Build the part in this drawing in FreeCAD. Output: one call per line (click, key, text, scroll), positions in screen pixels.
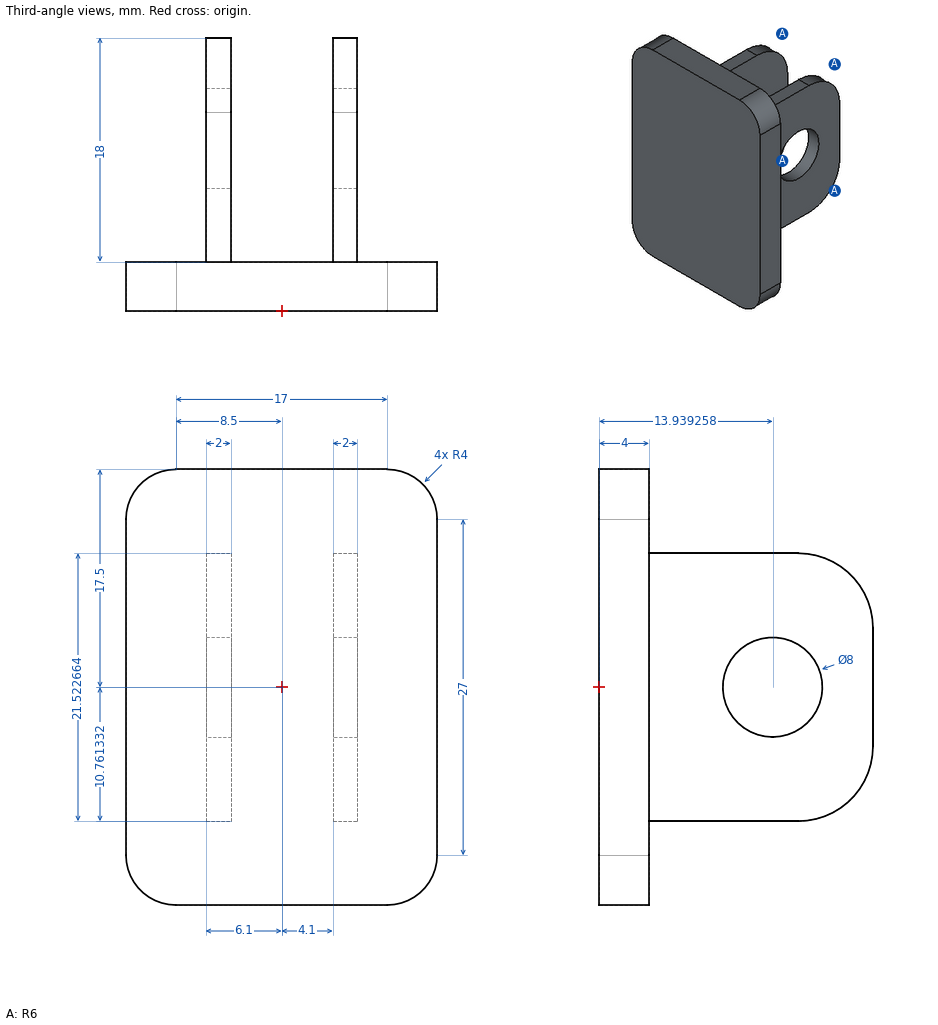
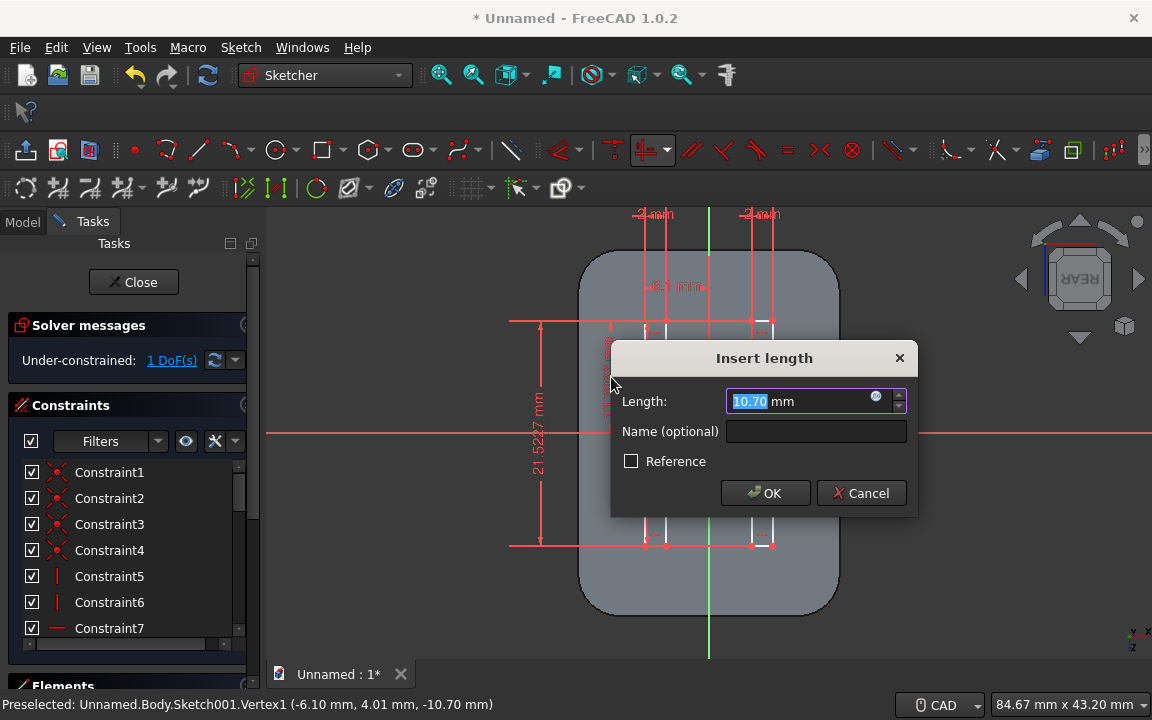
text(10.761332)
key(Return)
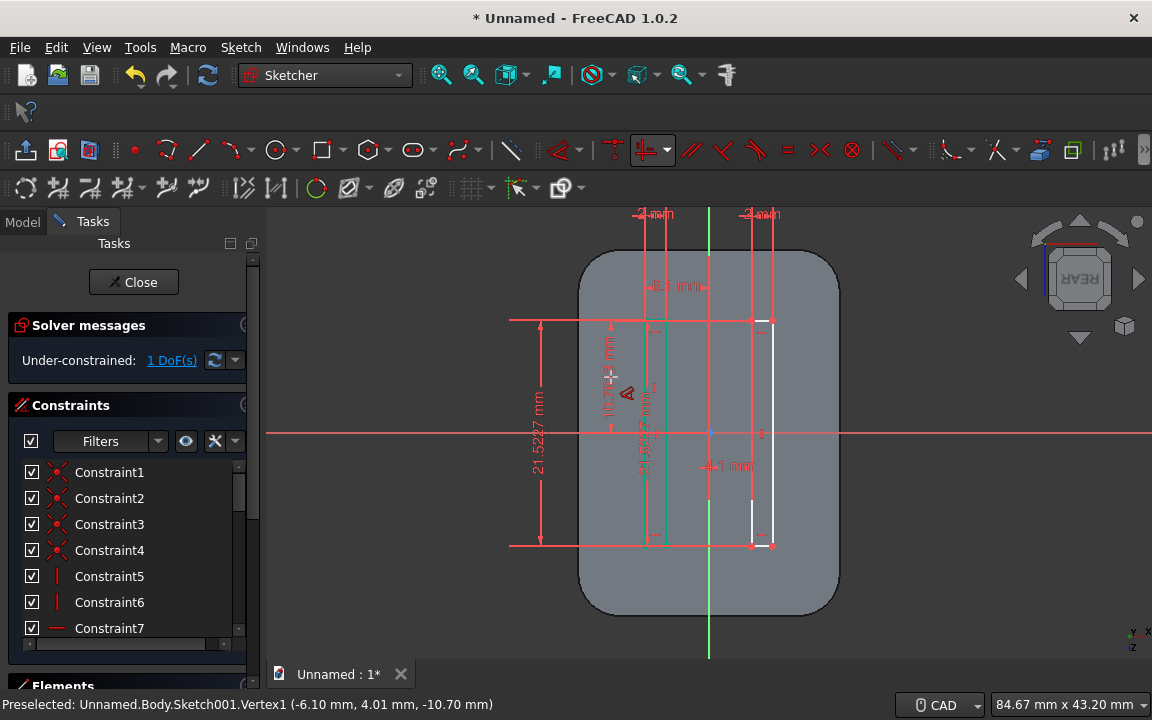
click(752, 321)
click(786, 377)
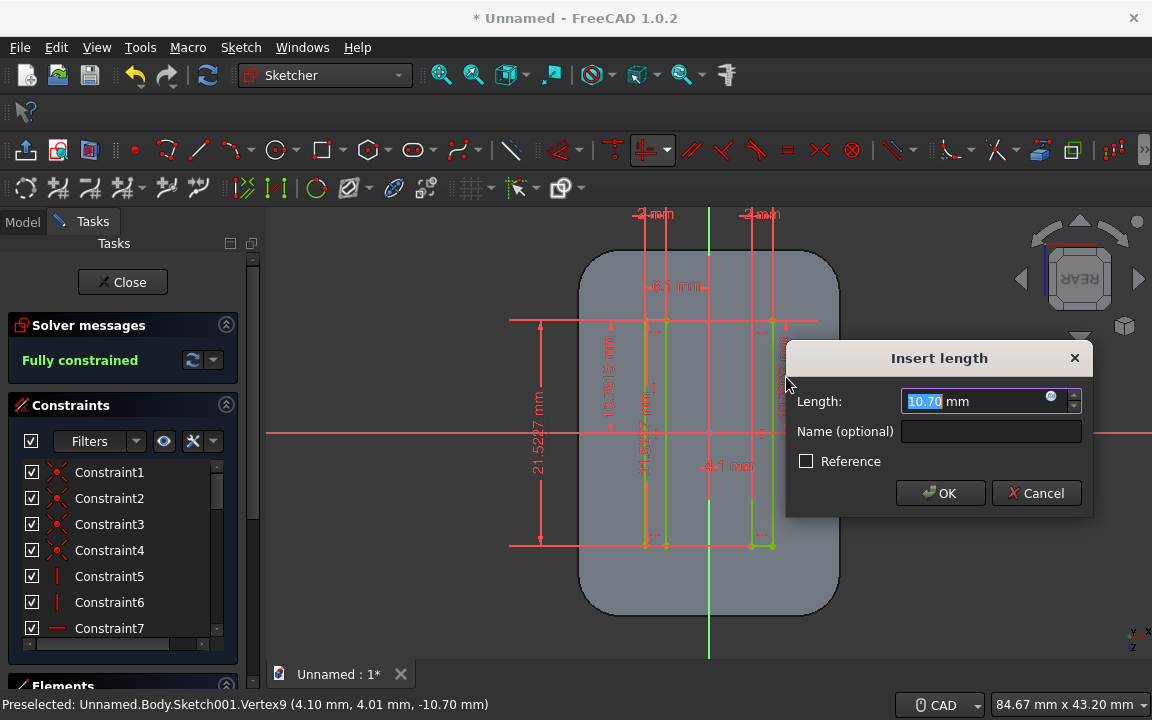
text(10.761332)
key(Return)
key(Escape)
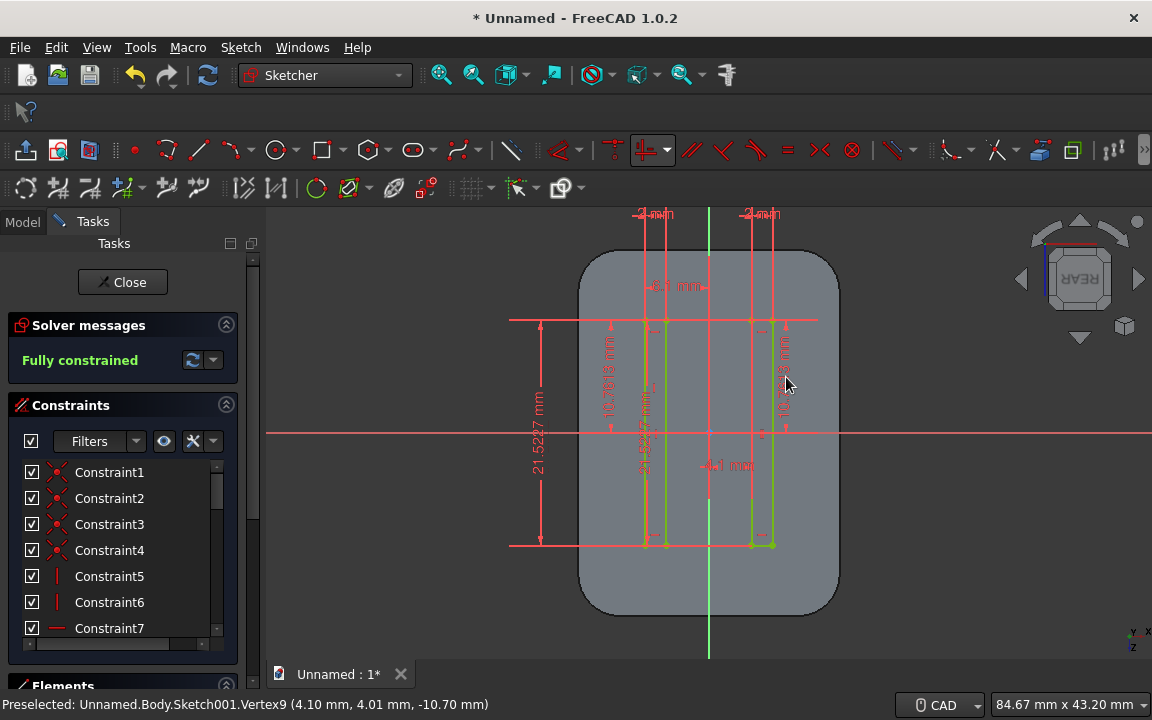
click(123, 282)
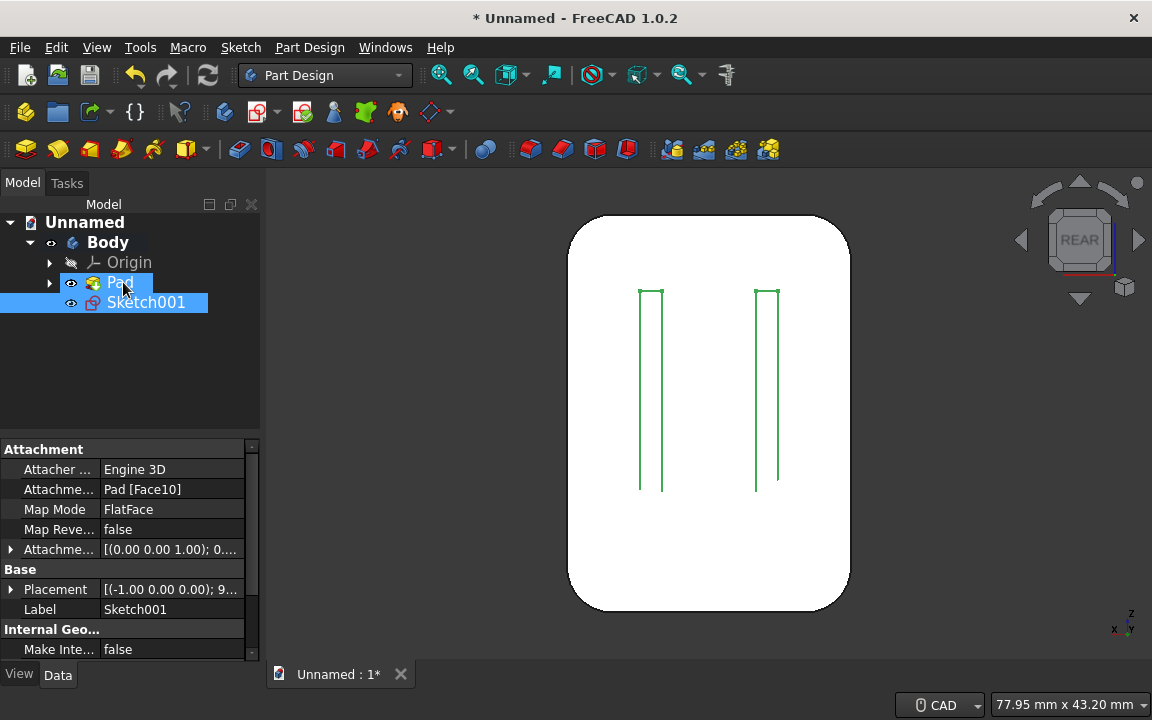
click(26, 150)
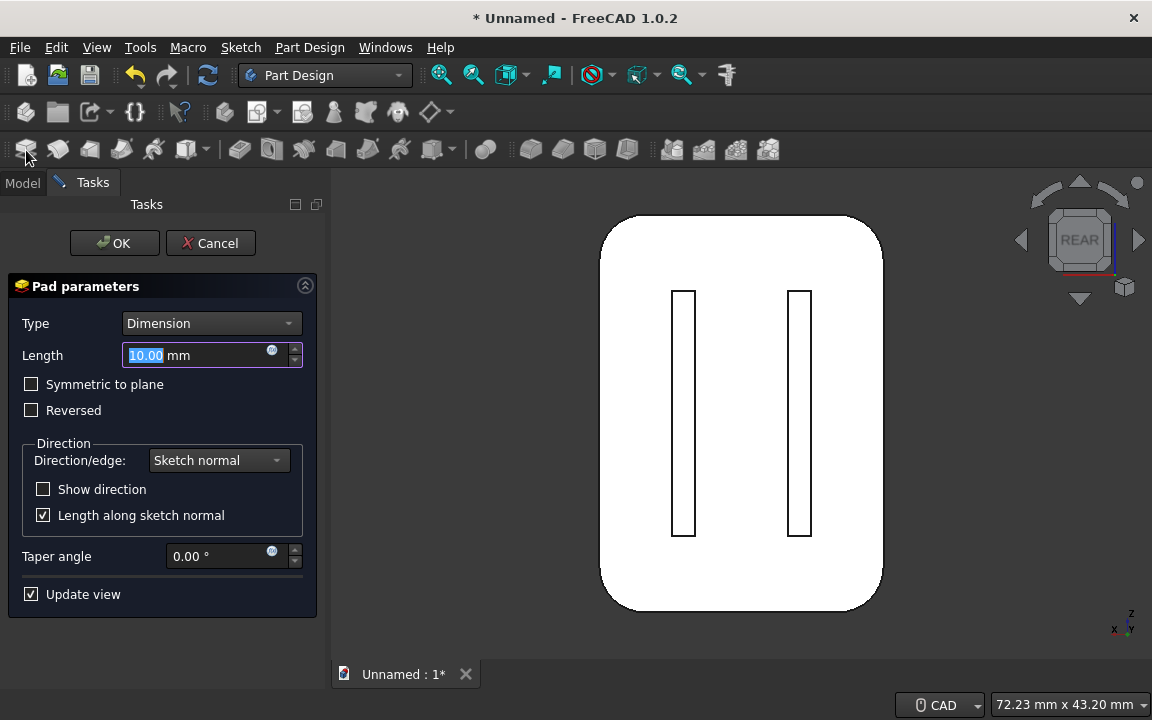
text(18)
key(Tab)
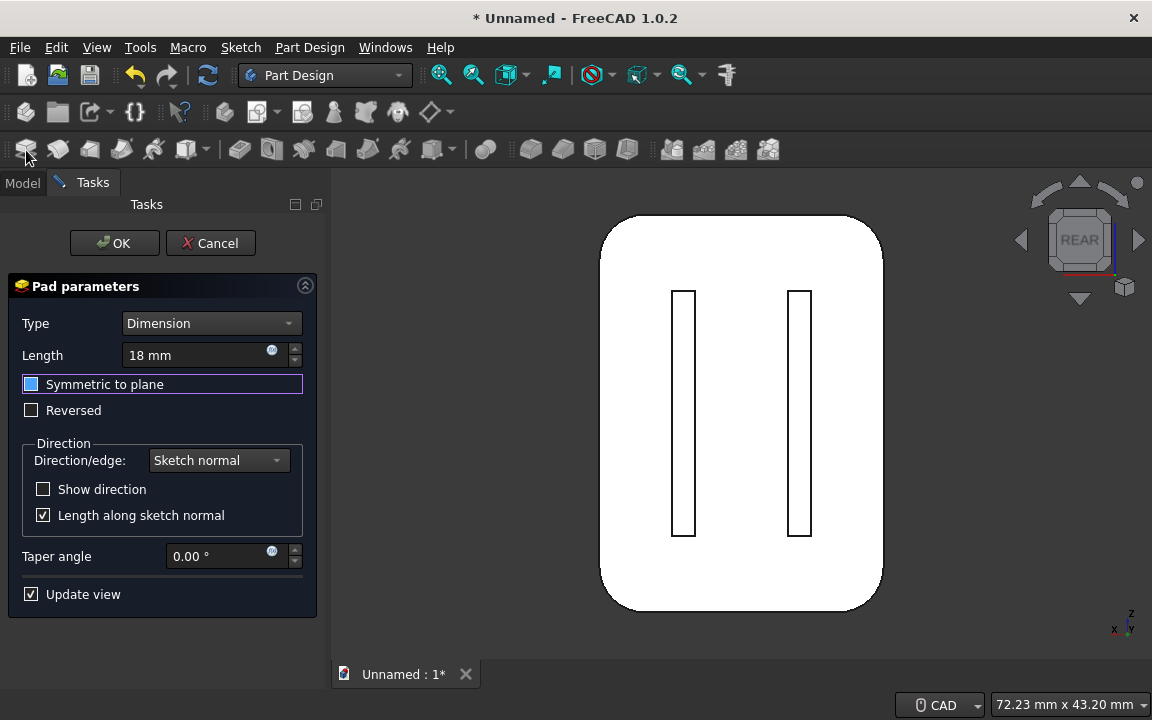
click(115, 243)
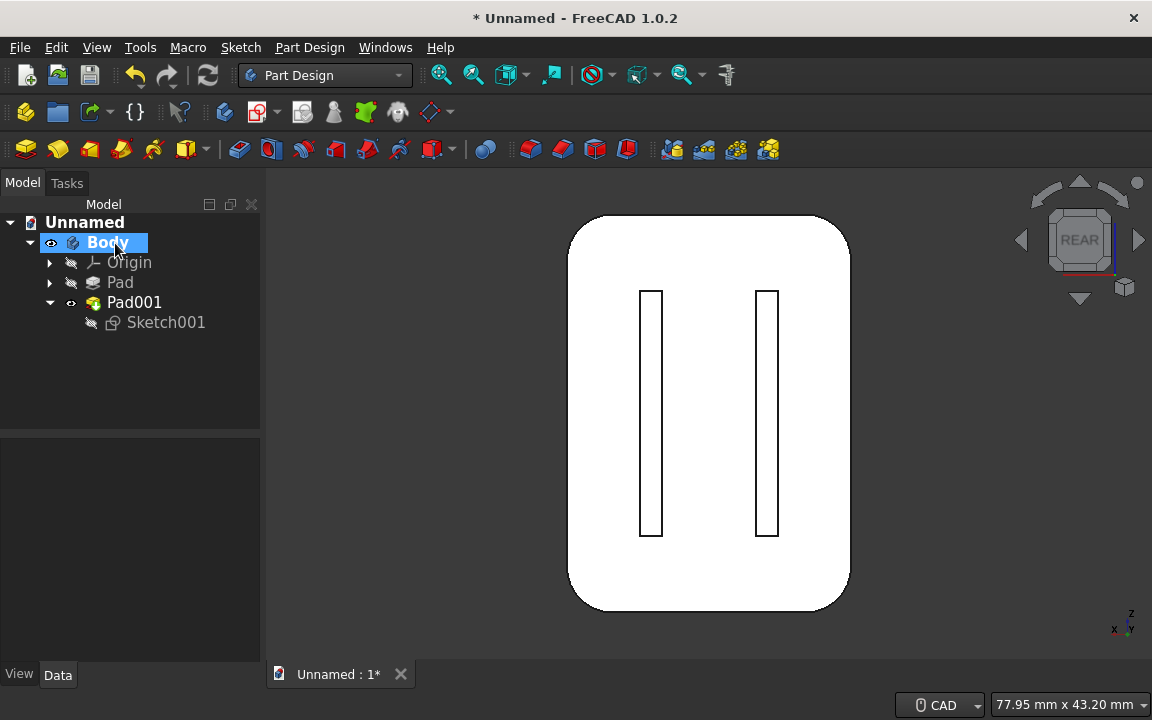
click(651, 535)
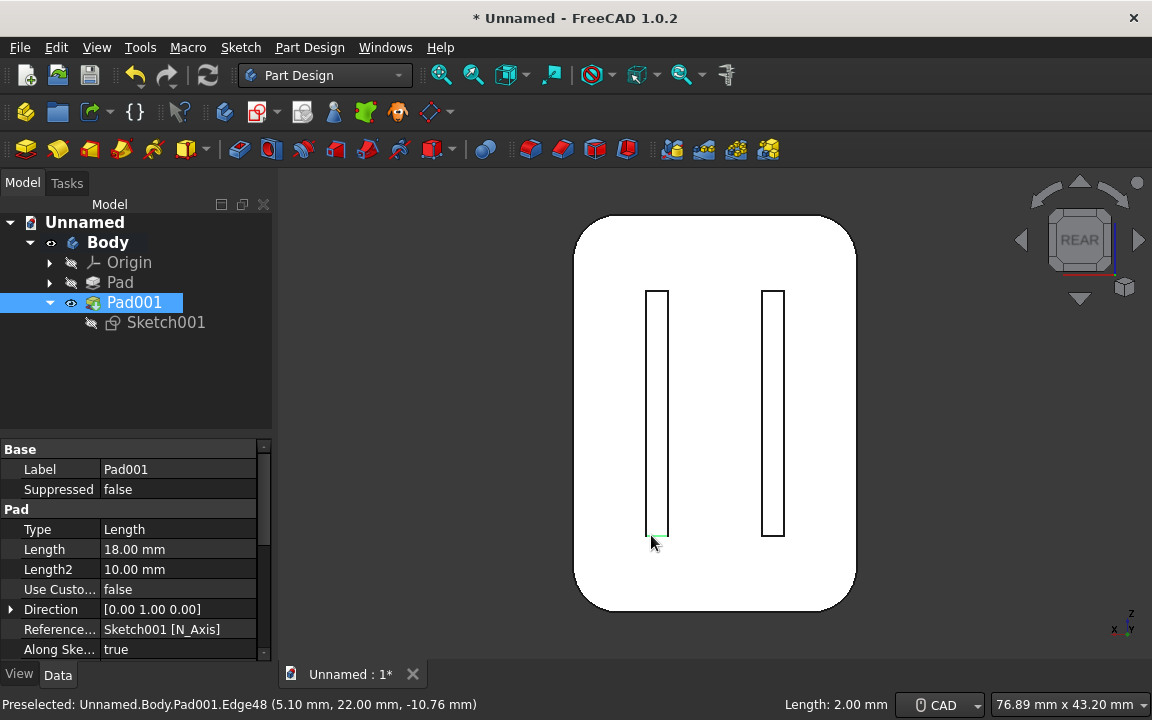
click(773, 535, ctrl)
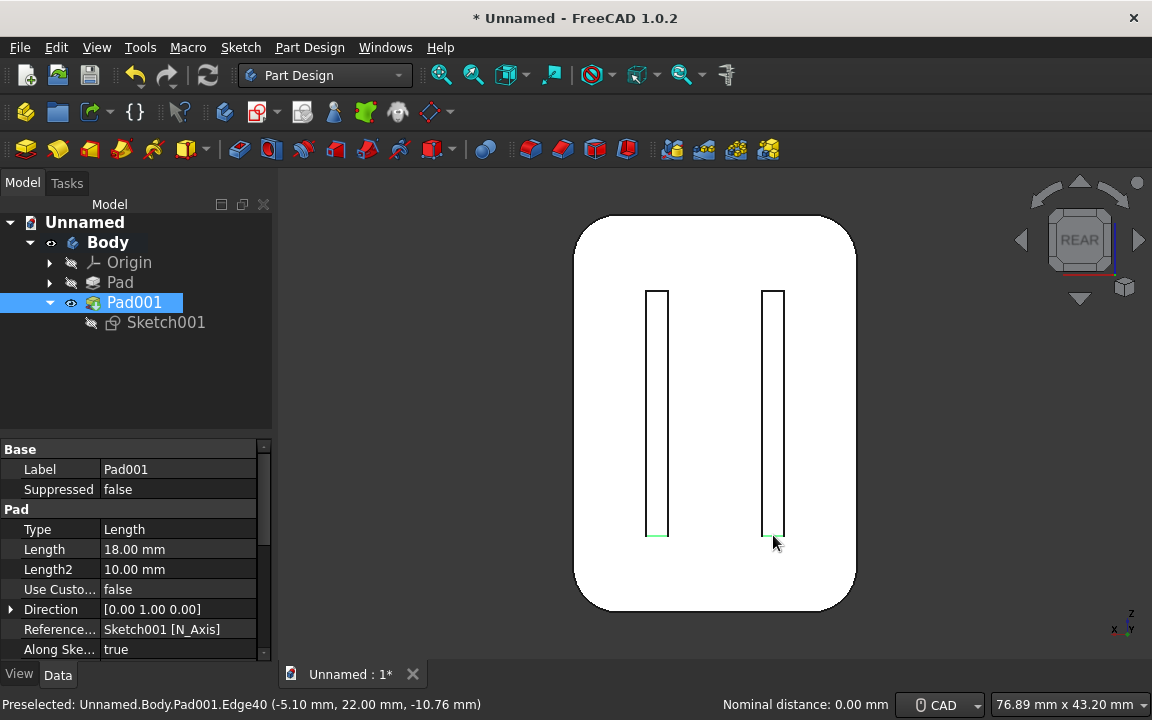
key(0)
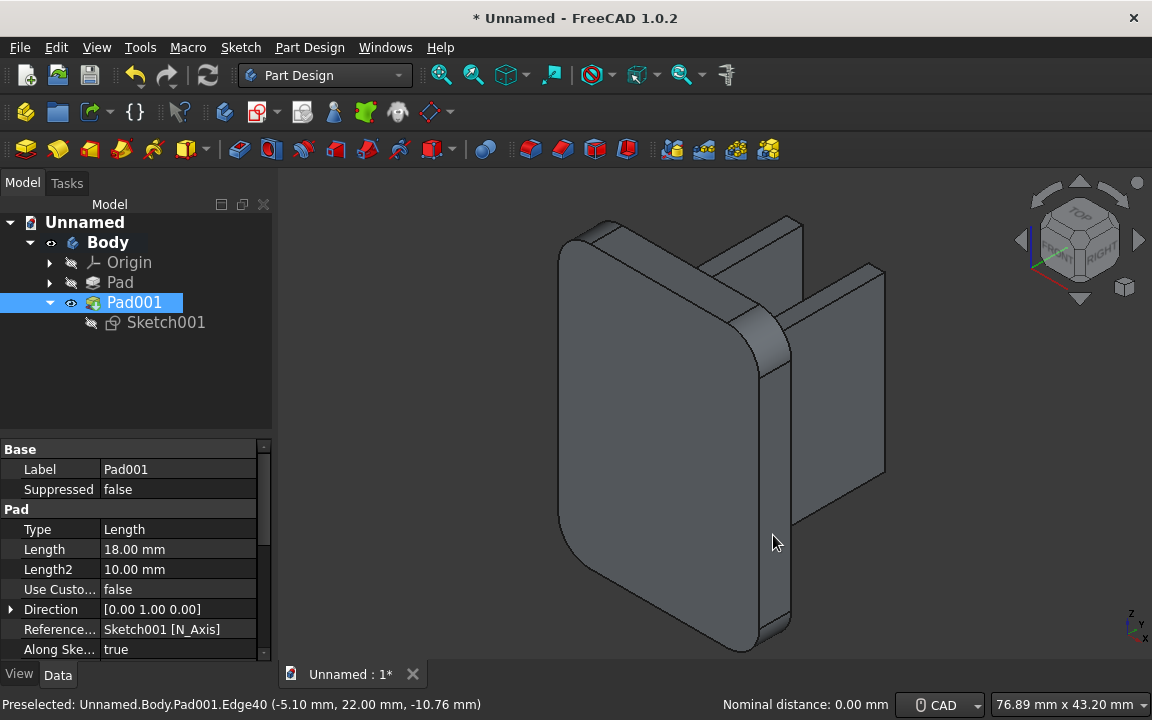
click(442, 76)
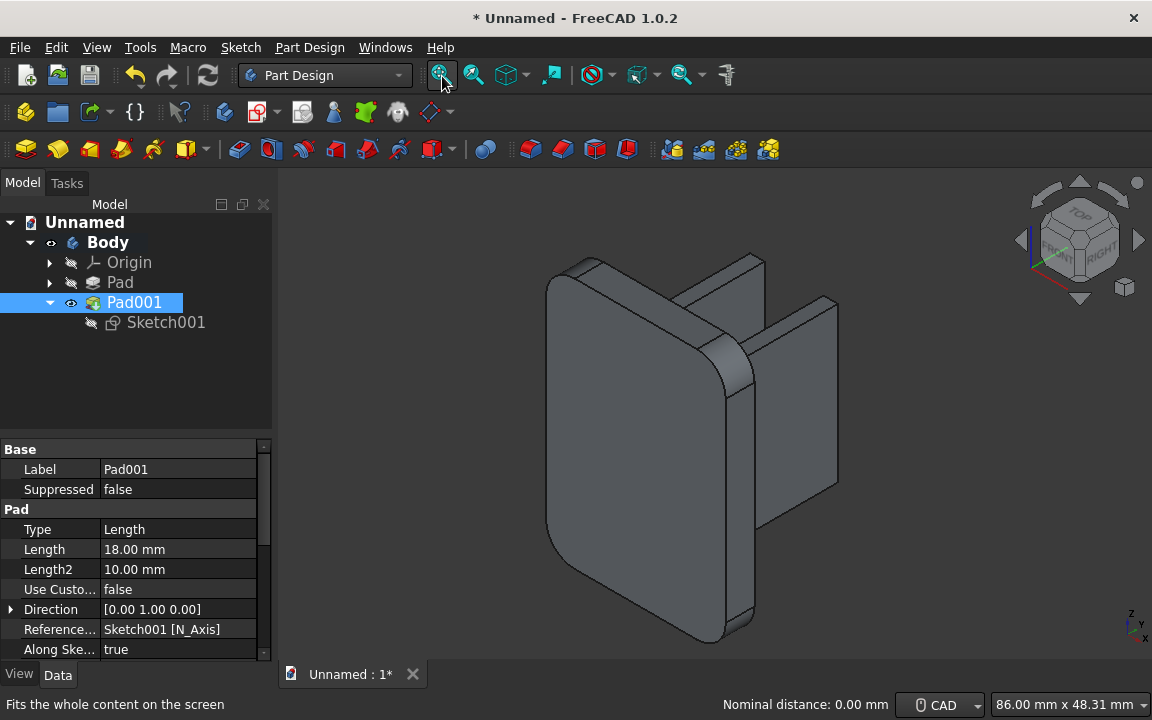
scroll(831, 299, up, 4)